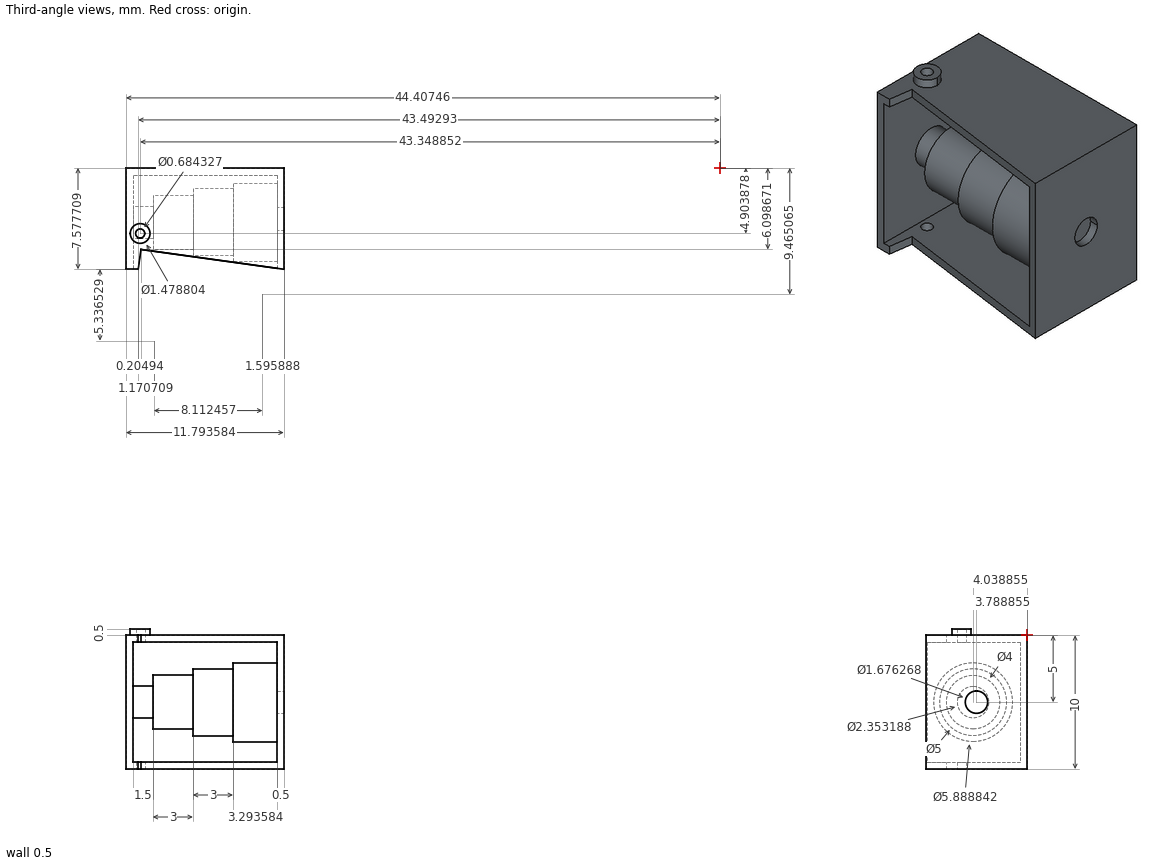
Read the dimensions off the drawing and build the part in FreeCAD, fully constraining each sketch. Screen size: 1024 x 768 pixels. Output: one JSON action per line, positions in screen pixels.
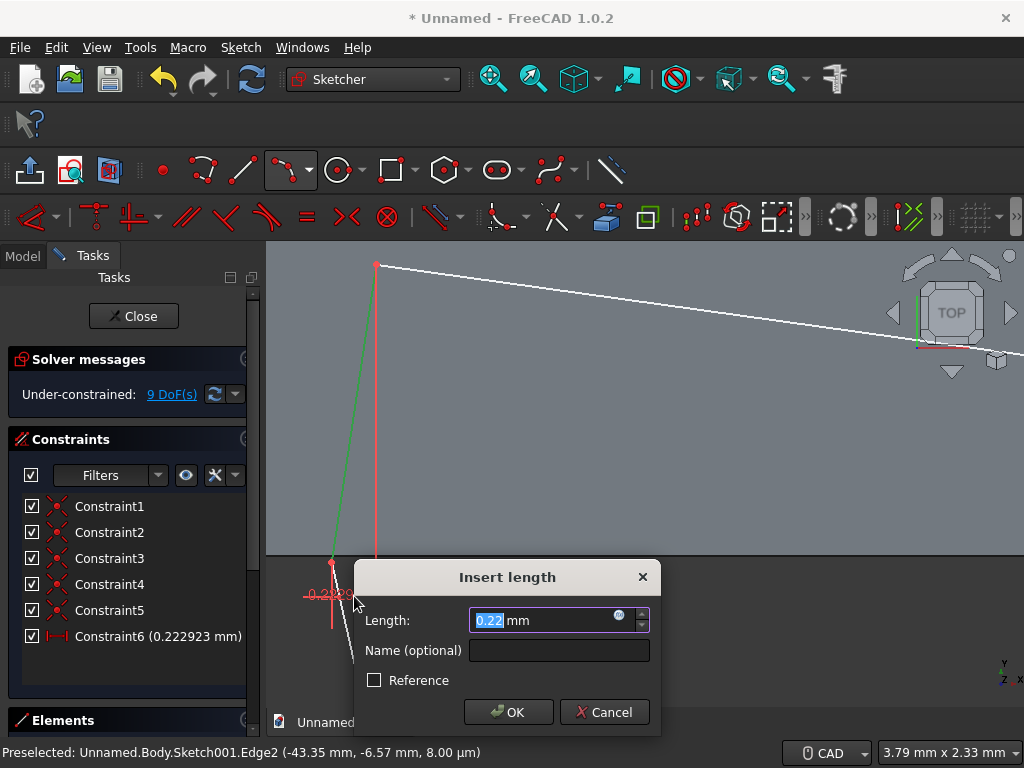
{"action": "type", "text": "0.20494"}
{"action": "key", "text": "Return"}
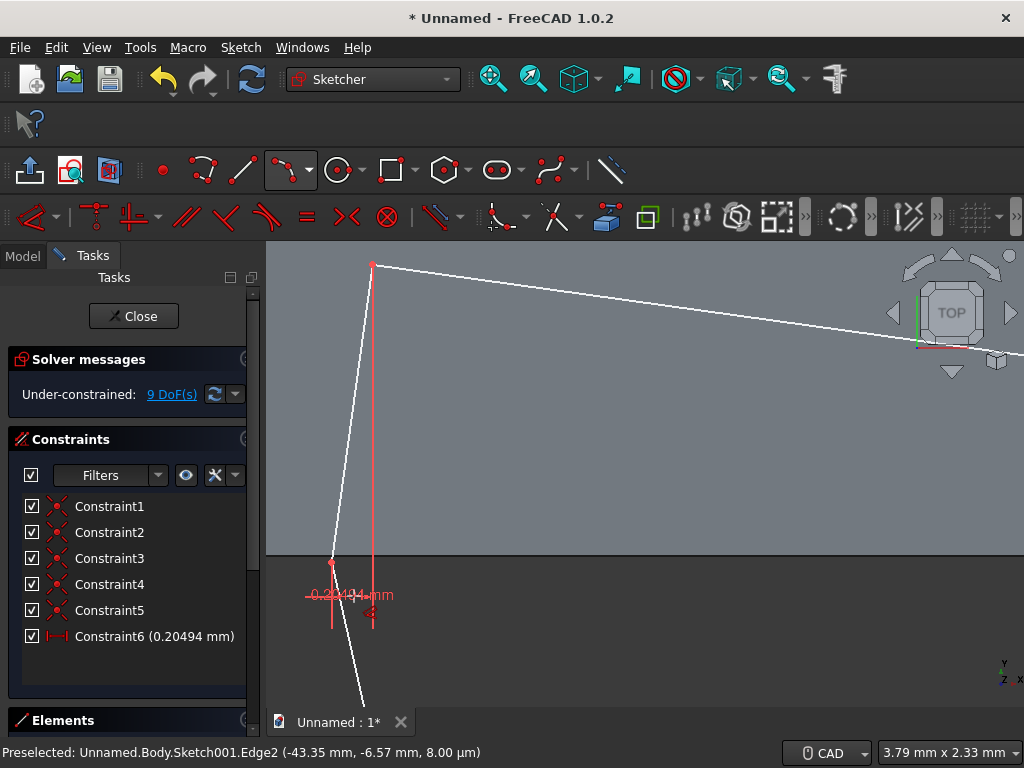
{"action": "scroll", "coordinate": [363, 356], "scroll_direction": "down", "scroll_amount": 8}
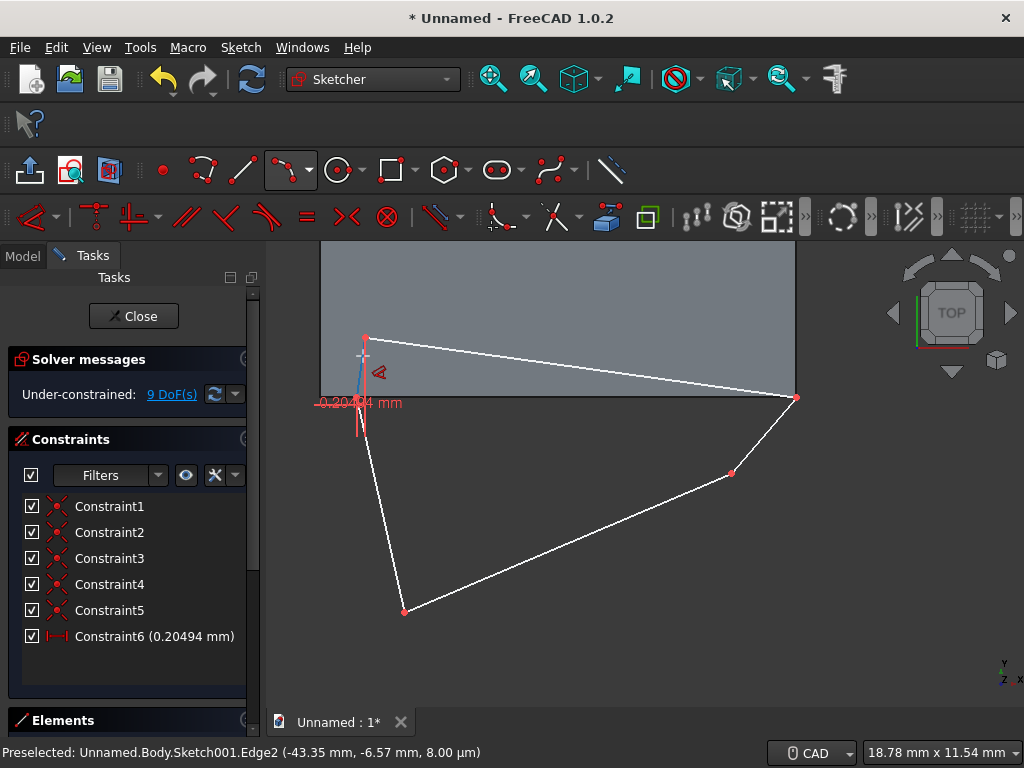
{"action": "left_click", "coordinate": [797, 398]}
{"action": "left_click", "coordinate": [763, 333]}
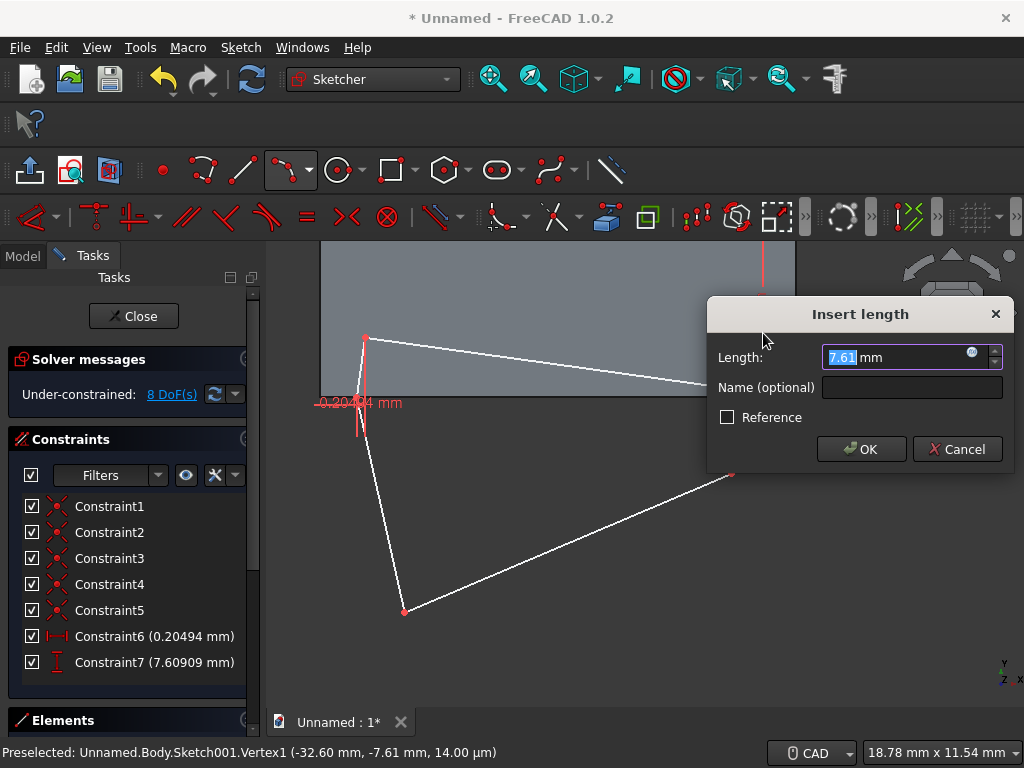
{"action": "type", "text": "7.577709"}
{"action": "key", "text": "Return"}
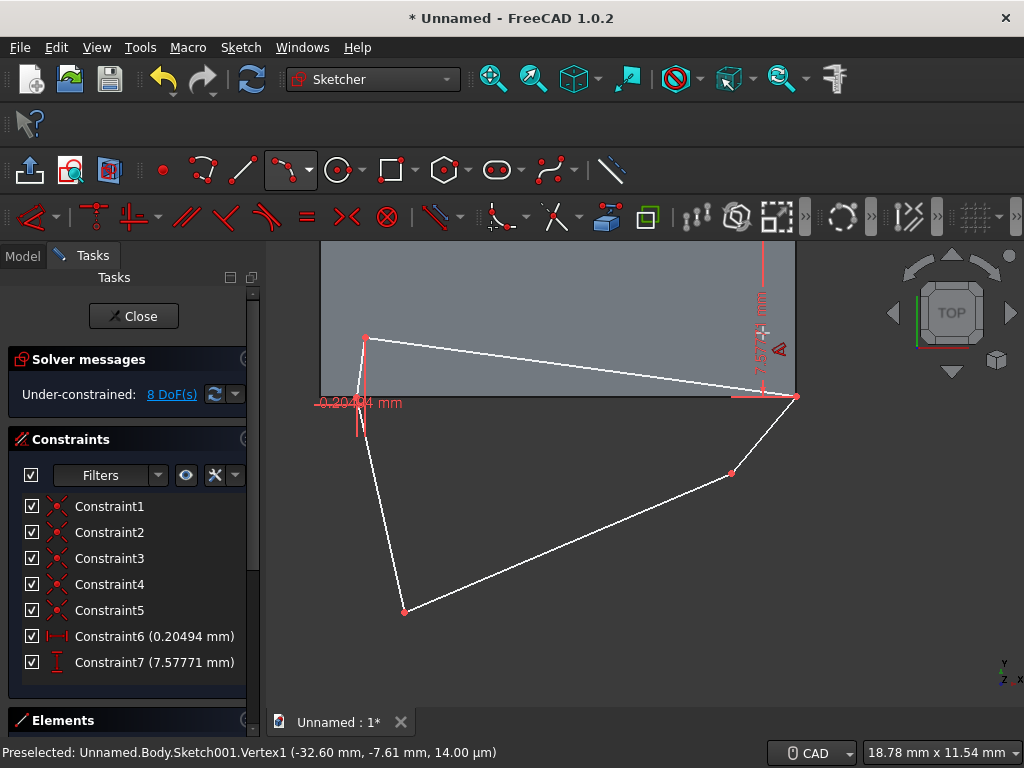
{"action": "left_click", "coordinate": [365, 338]}
{"action": "left_click", "coordinate": [331, 303]}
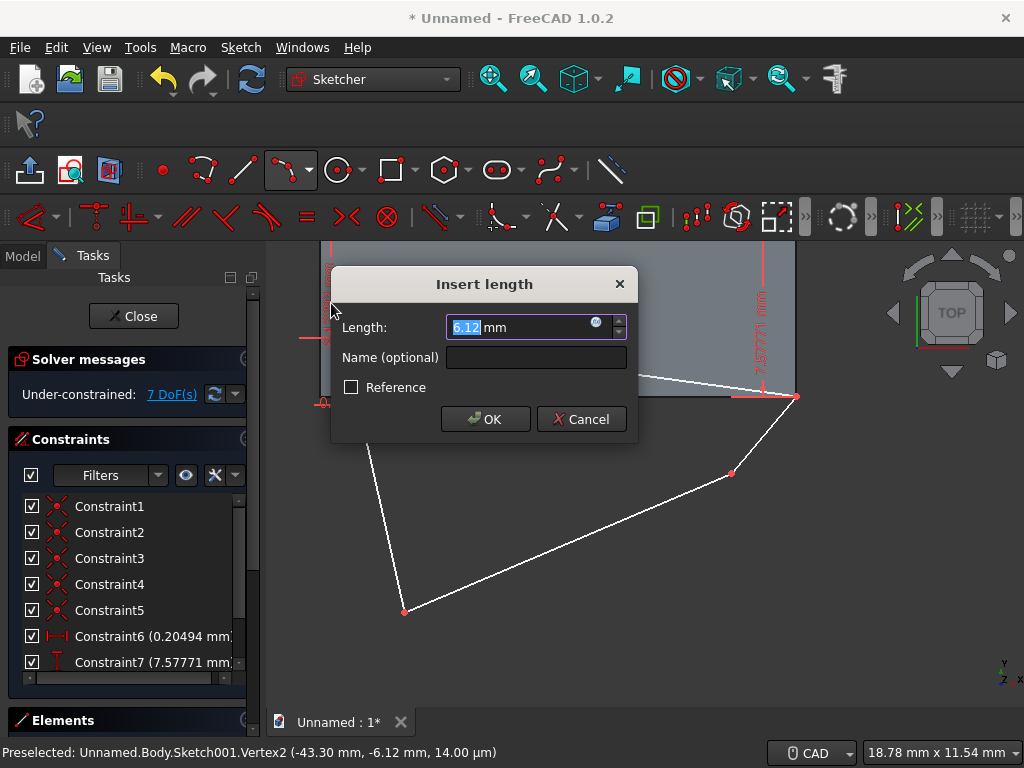
{"action": "type", "text": "6.098671"}
{"action": "key", "text": "Return"}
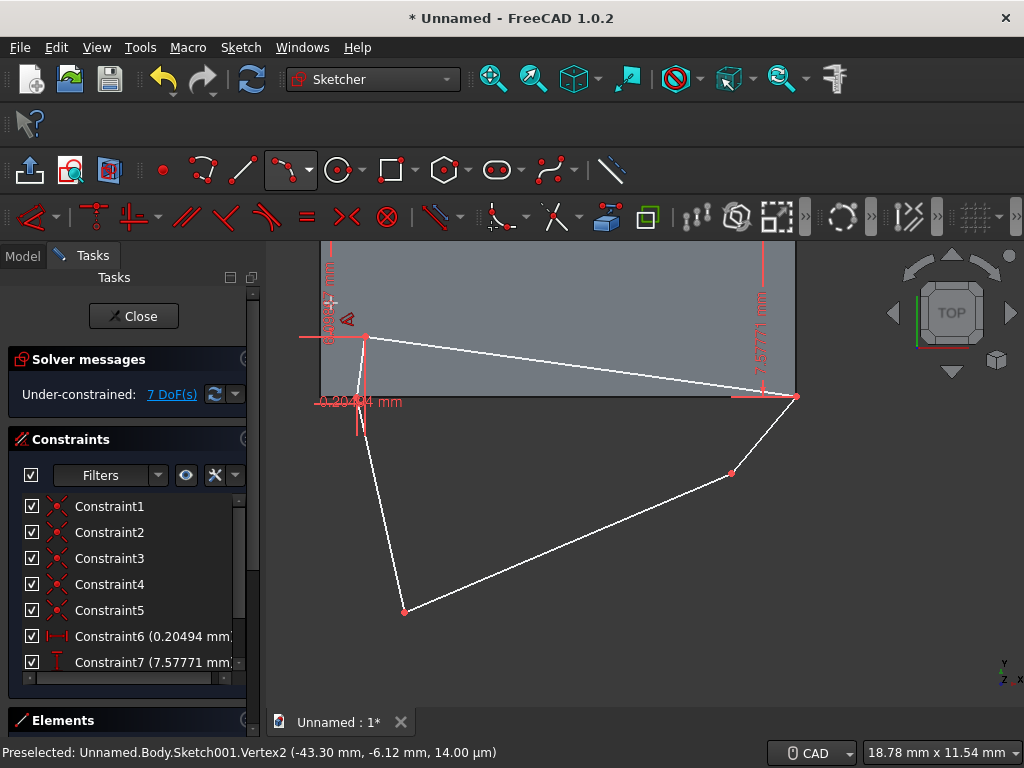
{"action": "left_click", "coordinate": [357, 398]}
{"action": "left_click", "coordinate": [608, 432]}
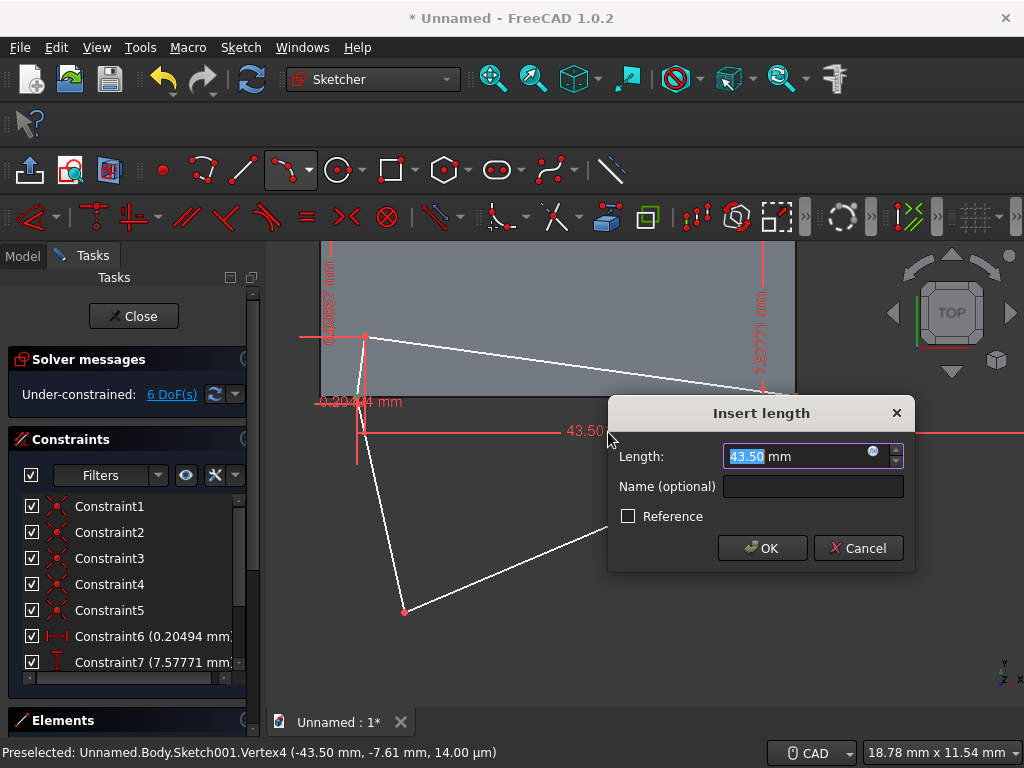
{"action": "type", "text": "43.49293"}
{"action": "key", "text": "Return"}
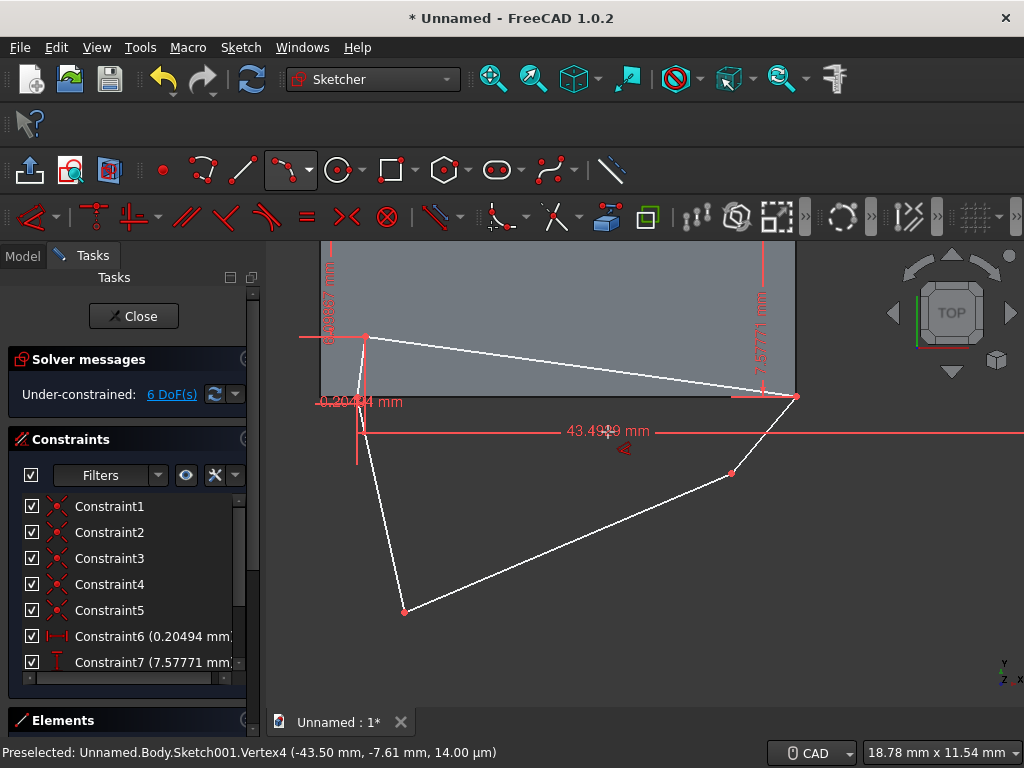
{"action": "left_click", "coordinate": [357, 398]}
{"action": "left_click", "coordinate": [323, 333]}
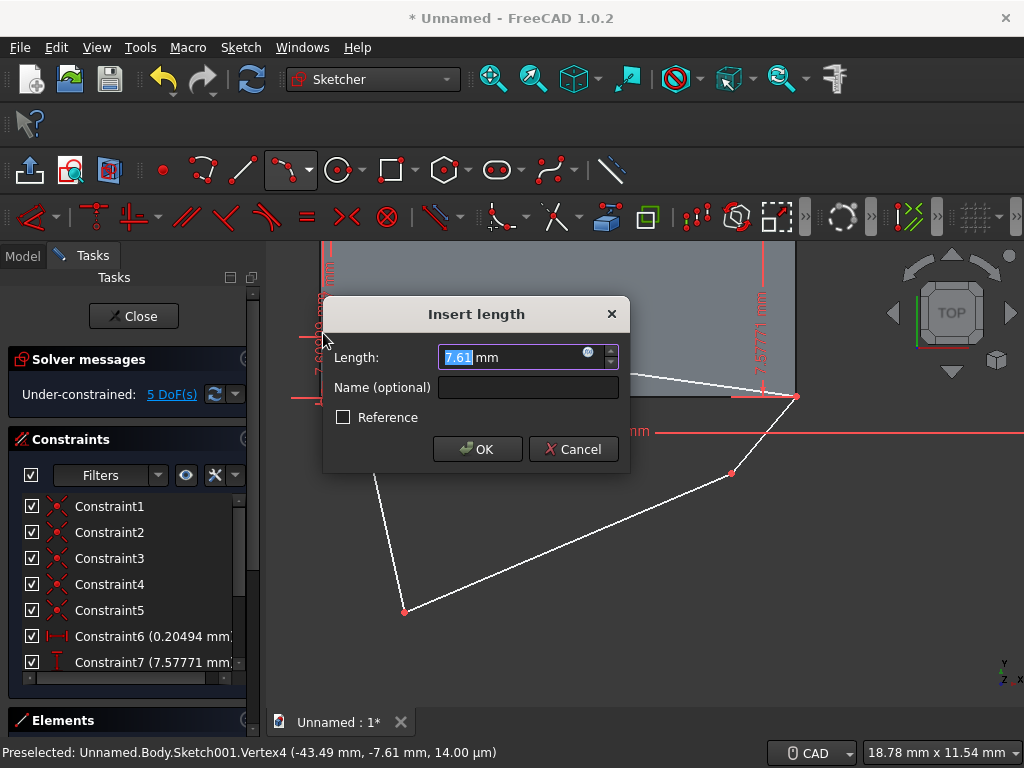
{"action": "type", "text": "7.577709"}
{"action": "key", "text": "Return"}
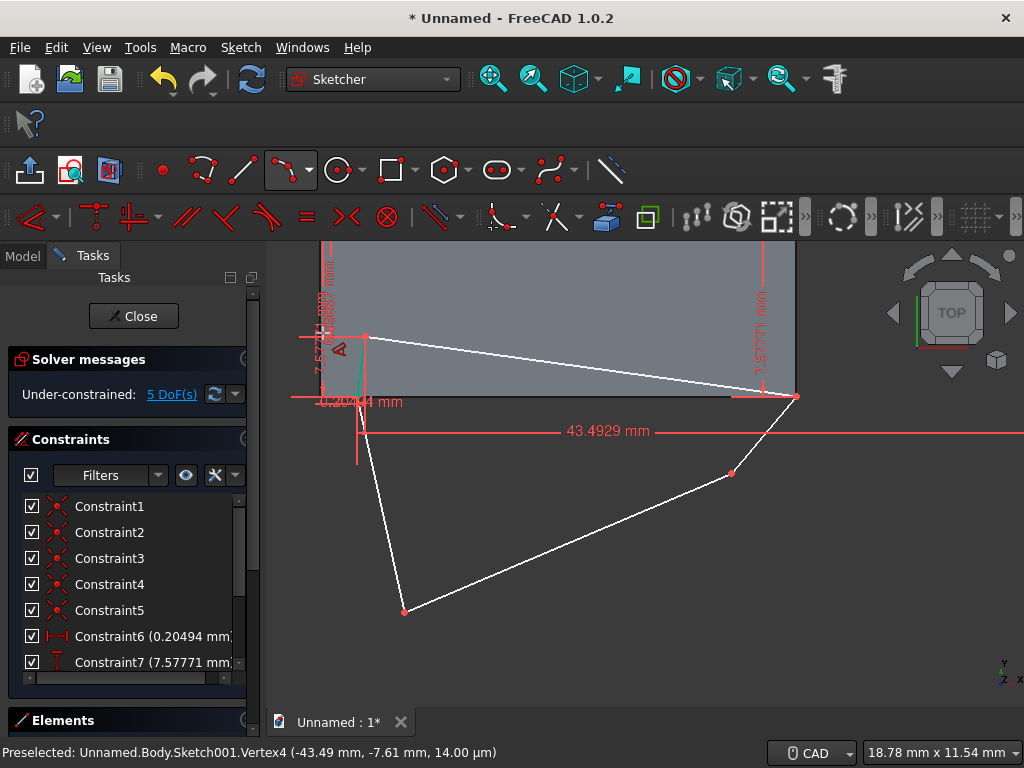
{"action": "left_click", "coordinate": [732, 474]}
{"action": "left_click", "coordinate": [698, 419]}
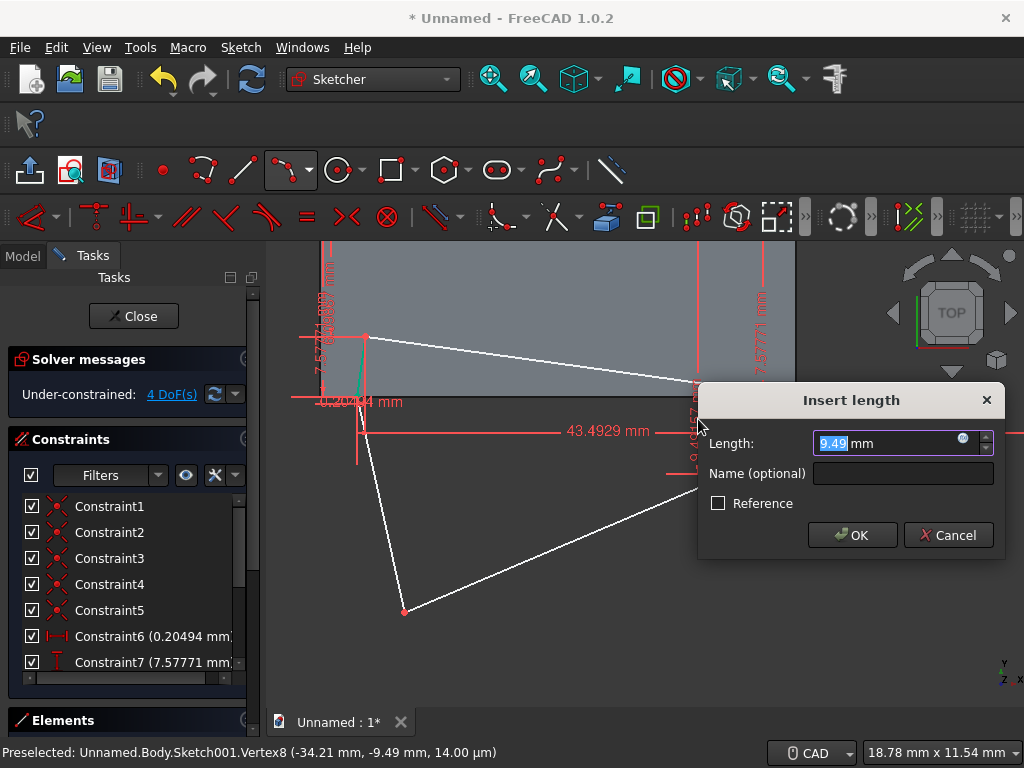
{"action": "type", "text": "9.465065"}
{"action": "key", "text": "Return"}